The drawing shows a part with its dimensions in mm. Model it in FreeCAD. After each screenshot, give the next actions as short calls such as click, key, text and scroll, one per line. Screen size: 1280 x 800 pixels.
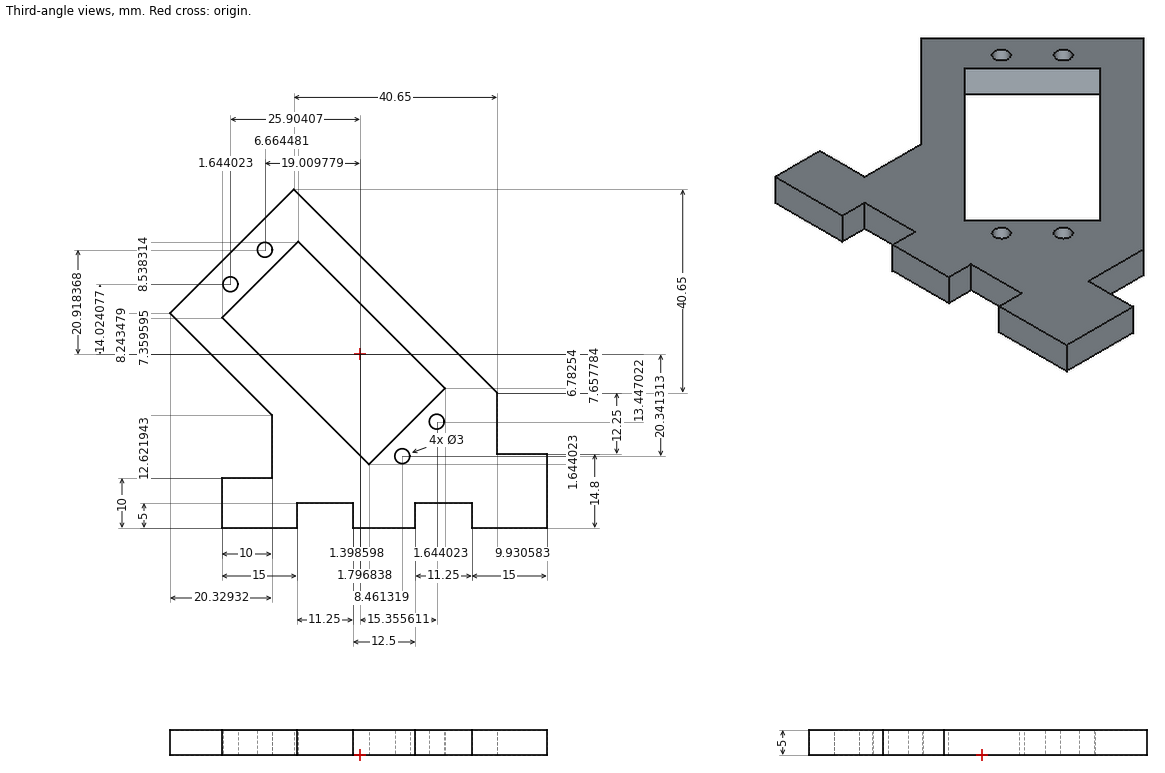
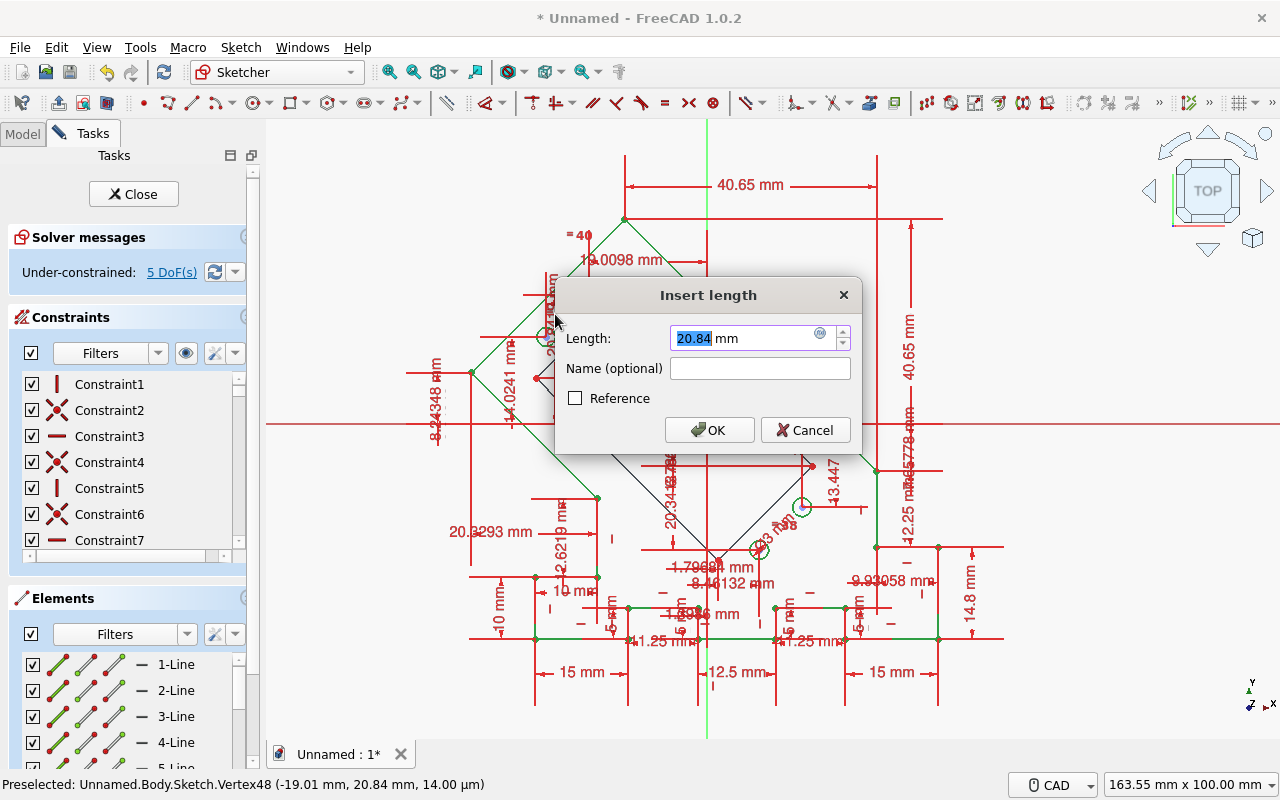
text(20.918368)
key(Return)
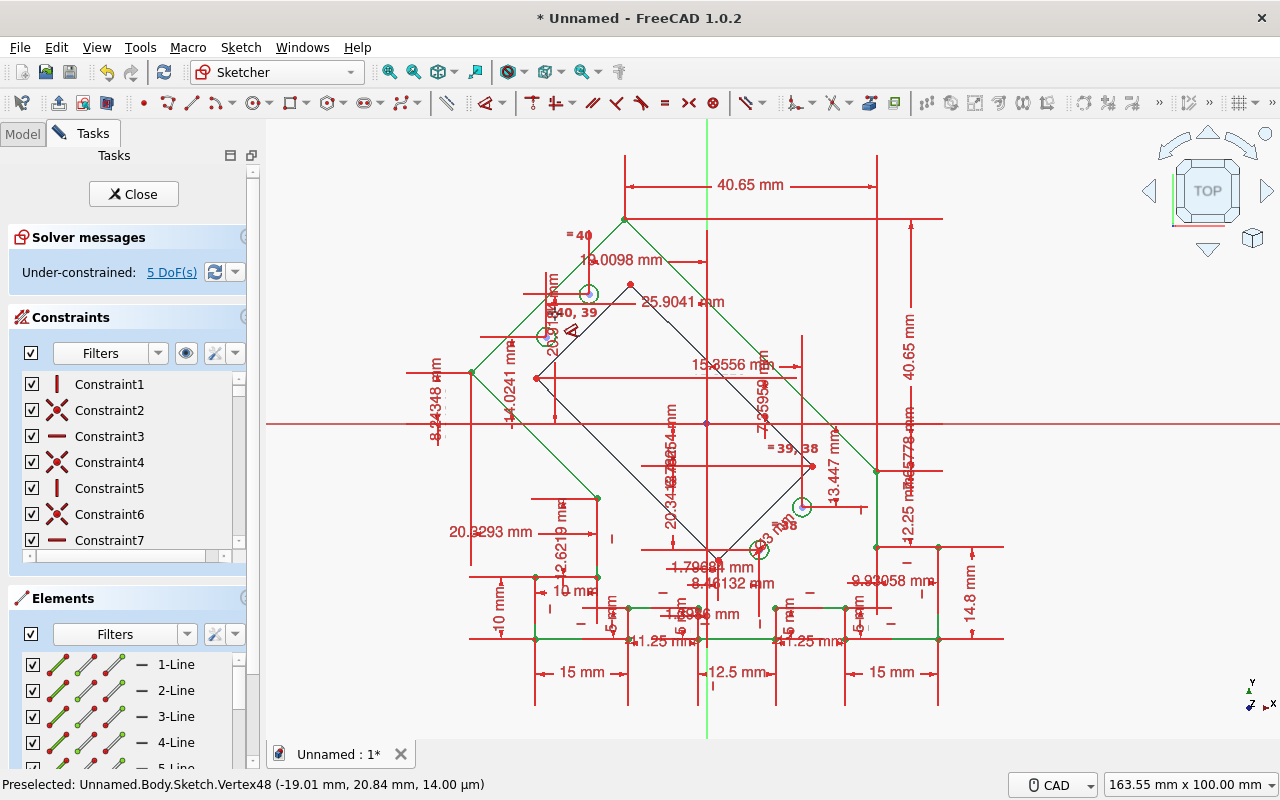
scroll(718, 561, up, 7)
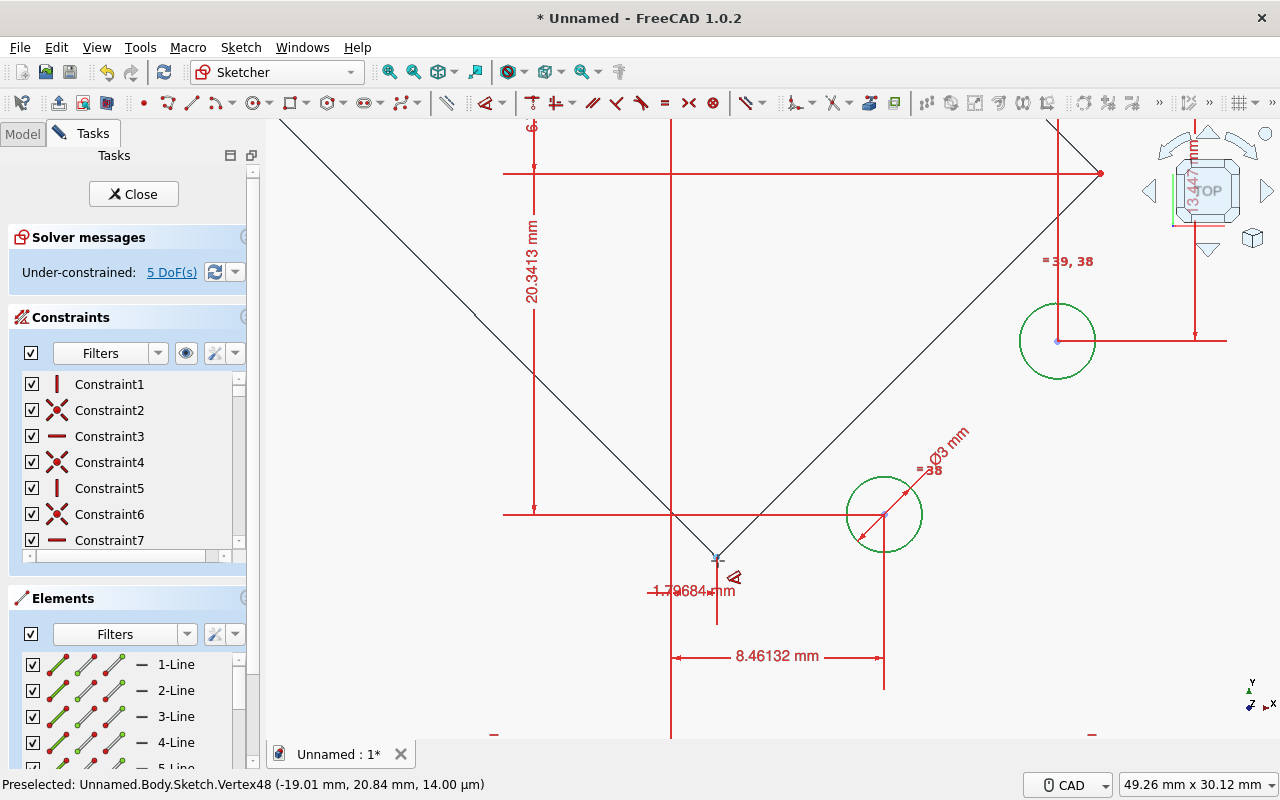
click(717, 558)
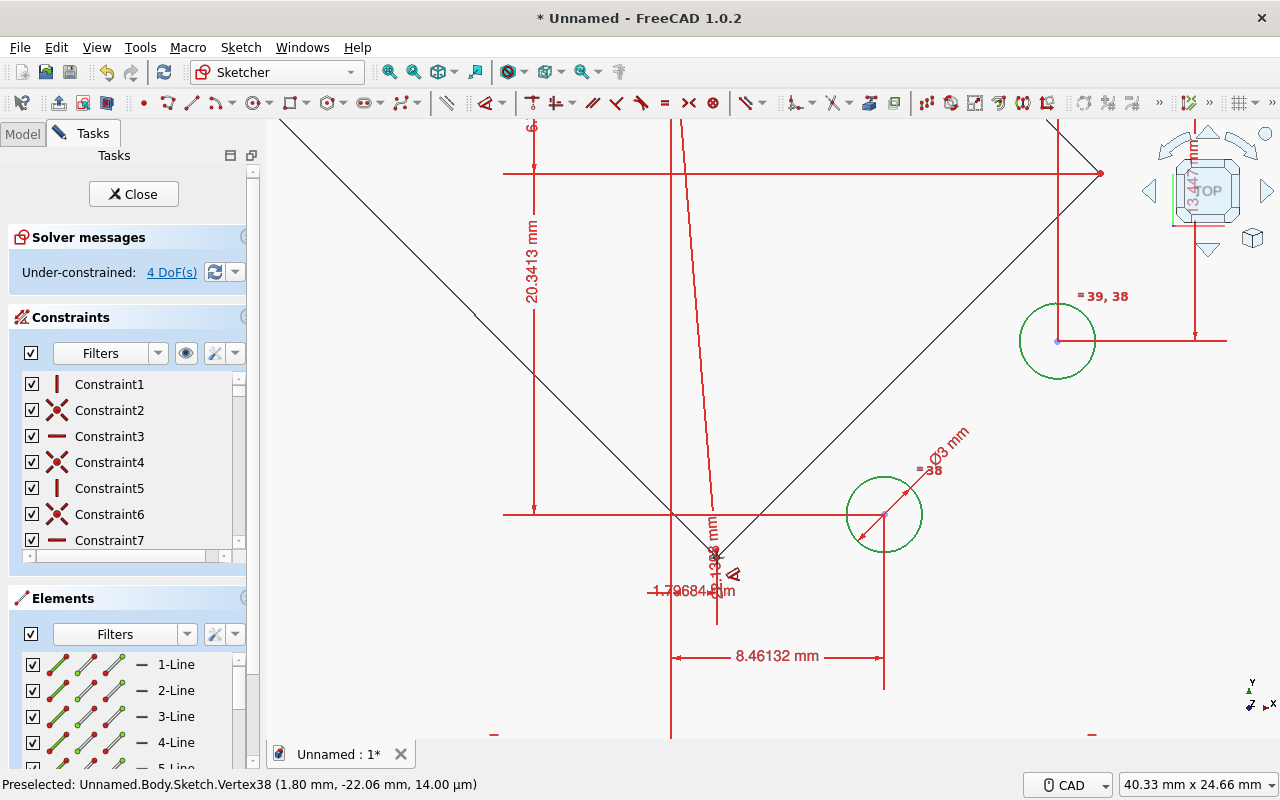
click(884, 515)
click(942, 536)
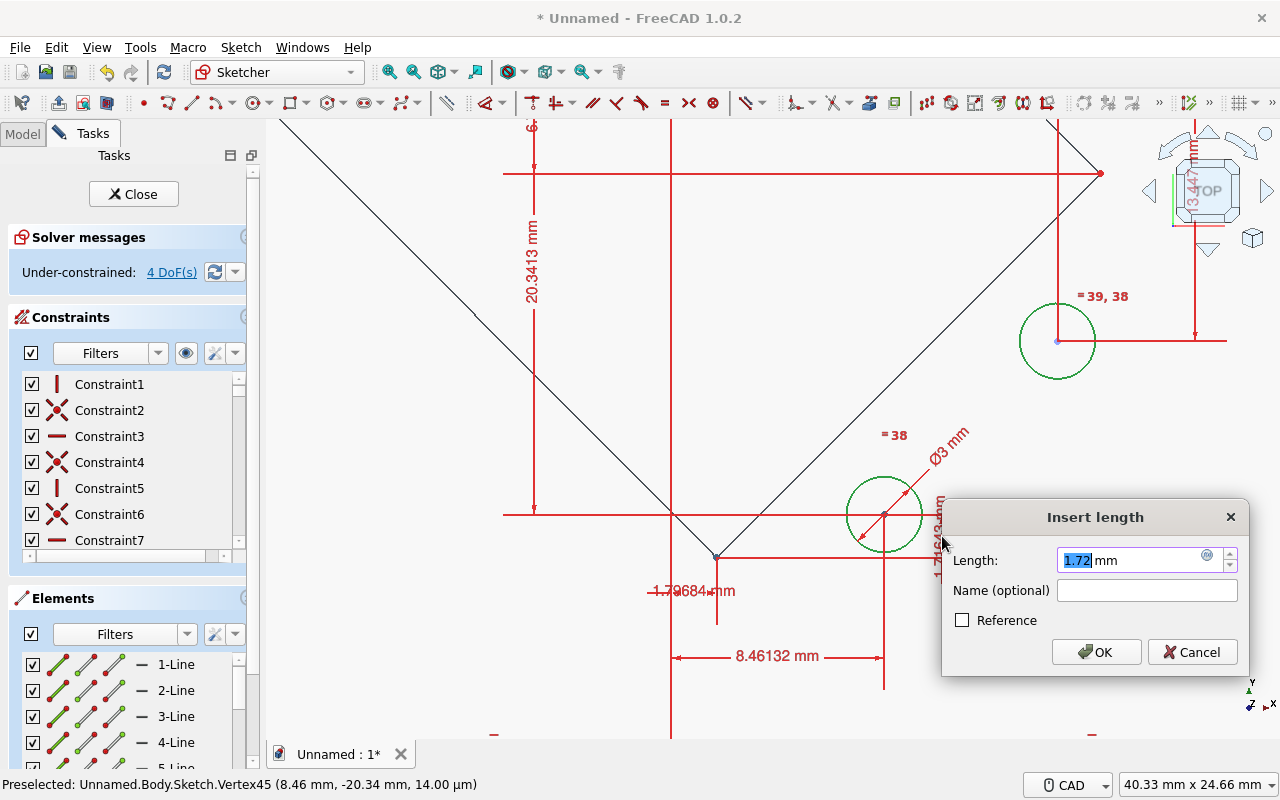
text(1.644023)
key(Return)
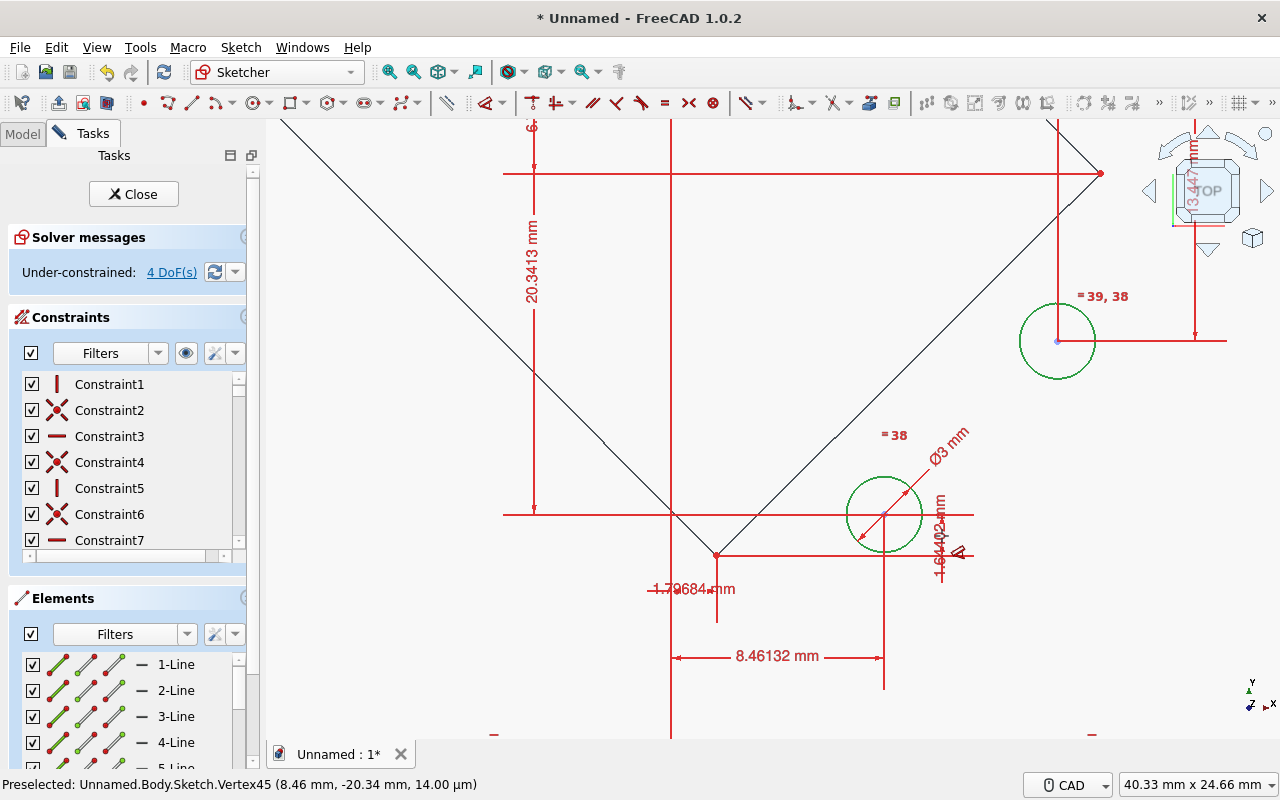
click(1101, 174)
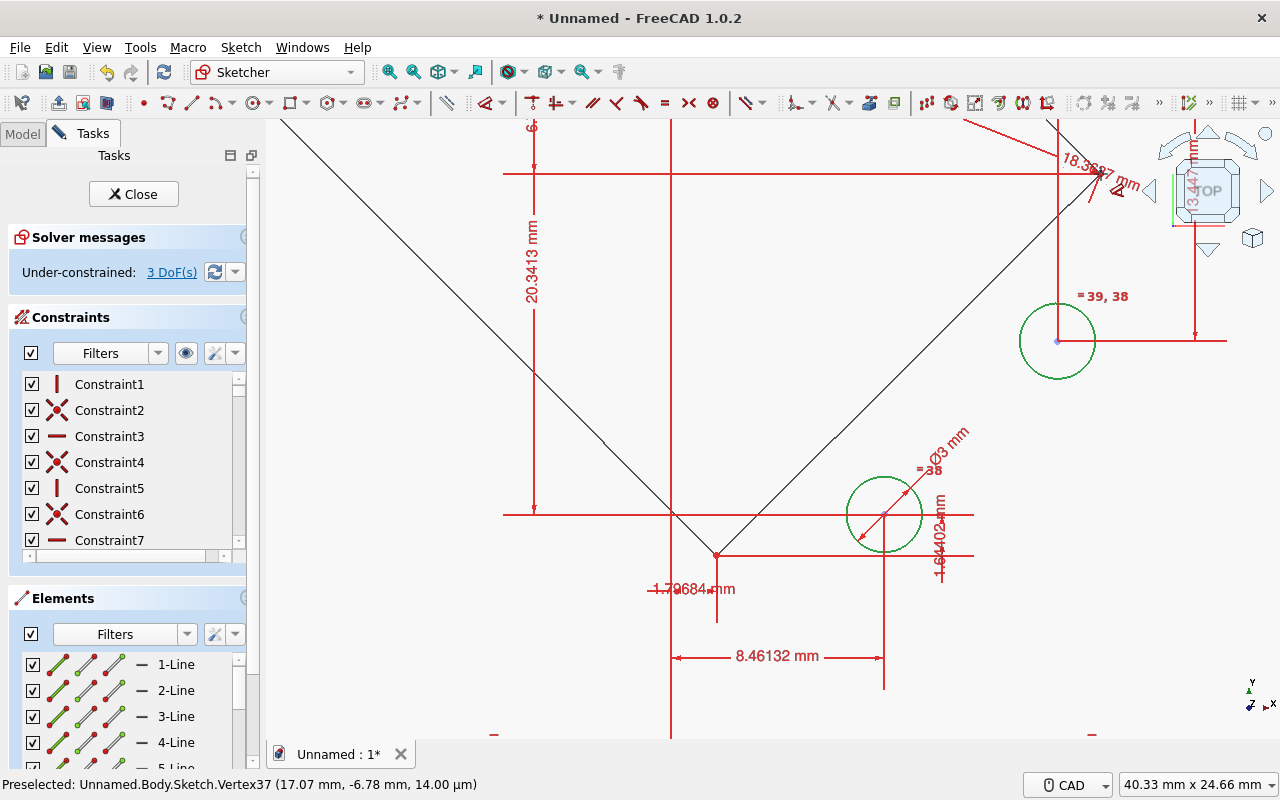
click(1058, 341)
click(1079, 399)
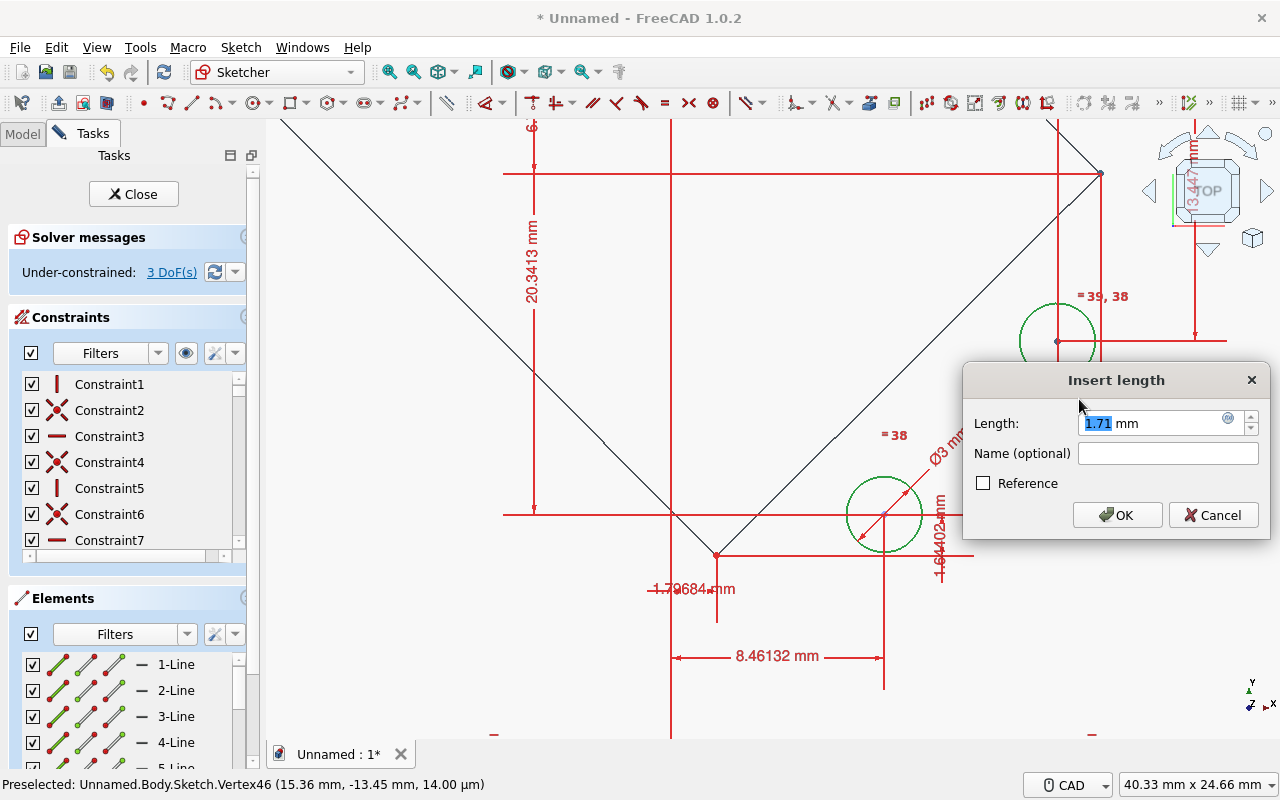
text(1.644023)
key(Return)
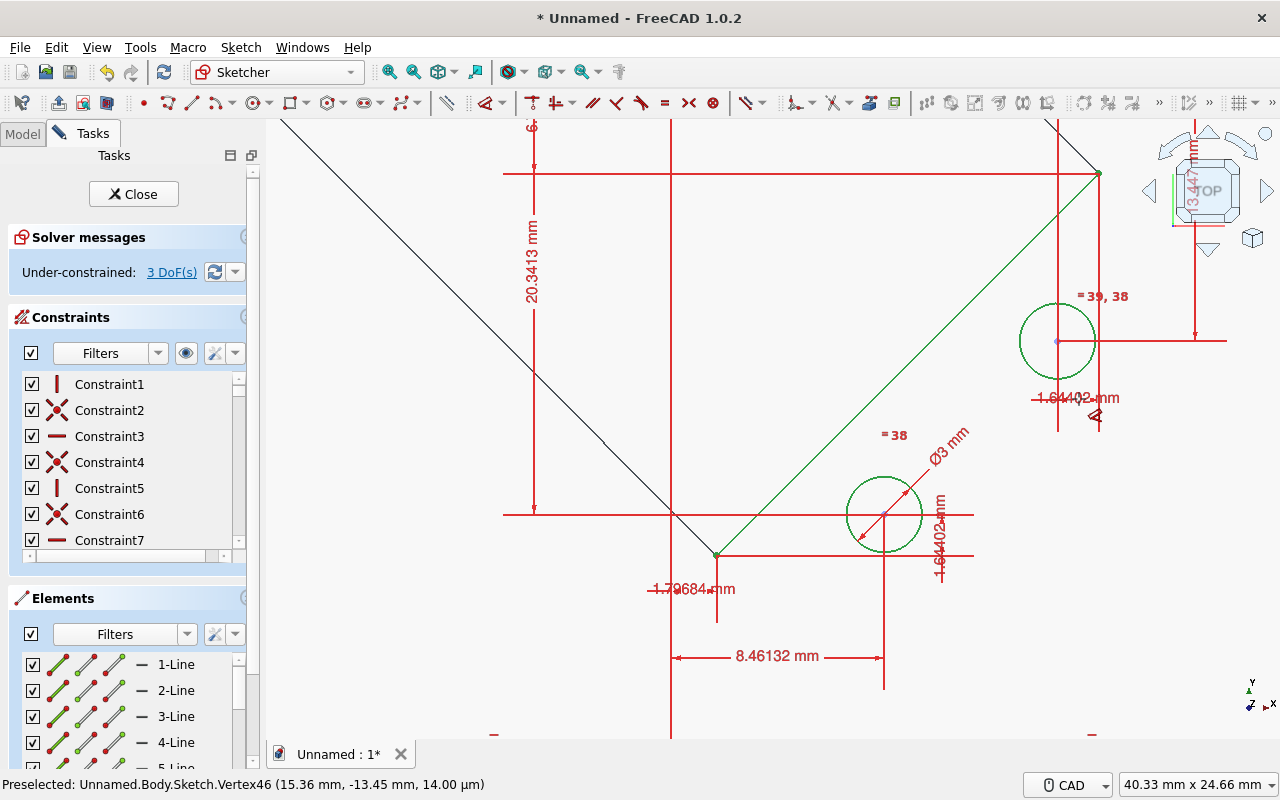
scroll(718, 561, down, 7)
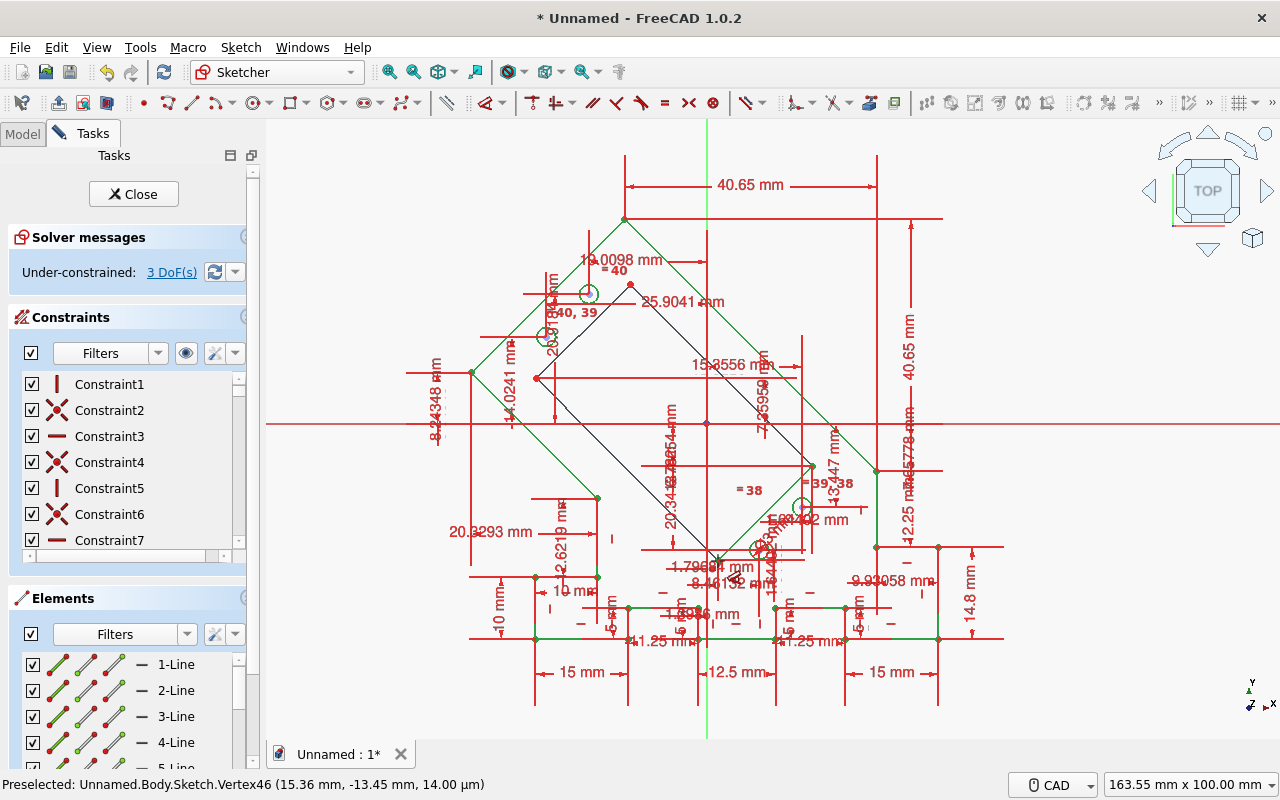
scroll(536, 378, up, 7)